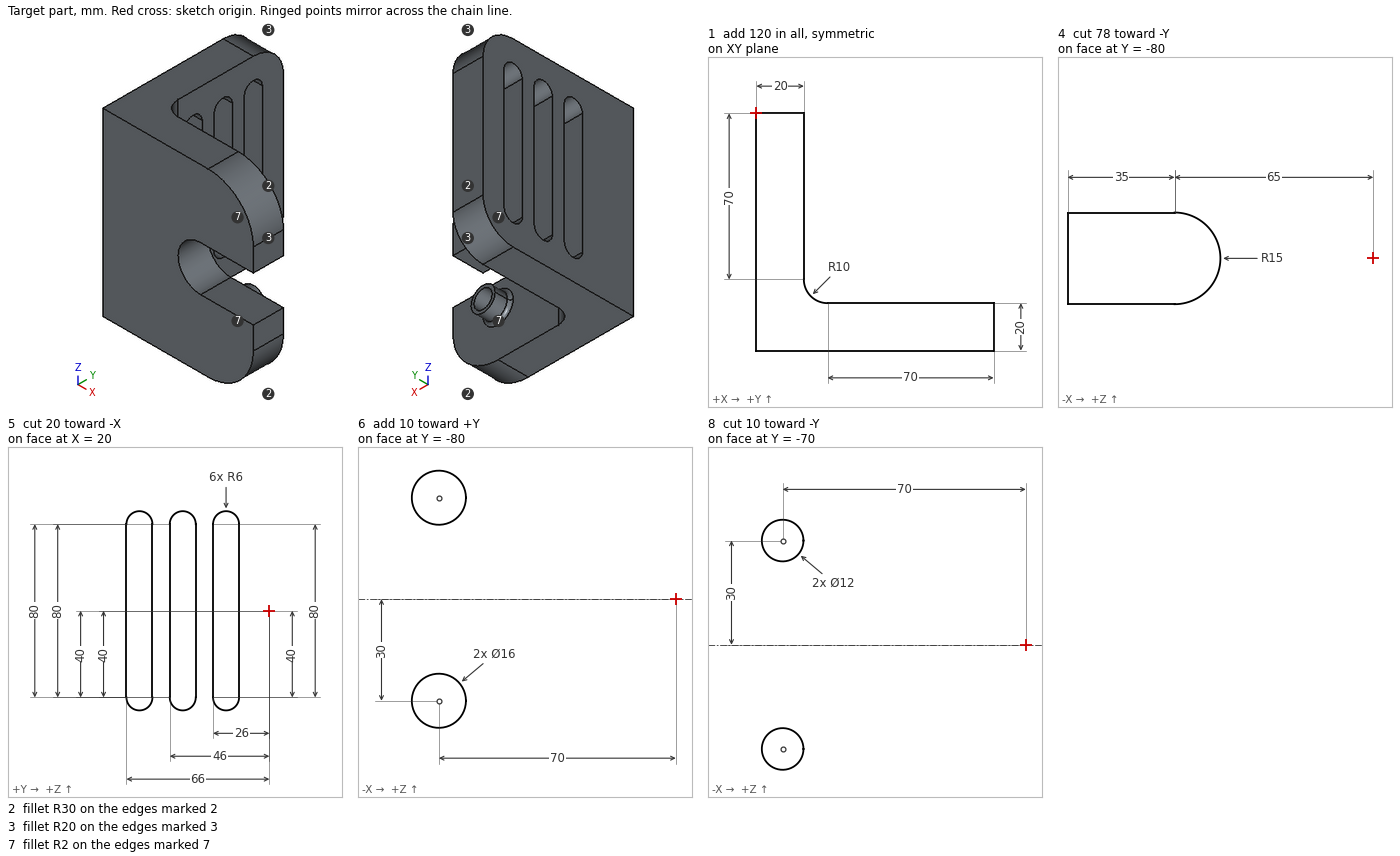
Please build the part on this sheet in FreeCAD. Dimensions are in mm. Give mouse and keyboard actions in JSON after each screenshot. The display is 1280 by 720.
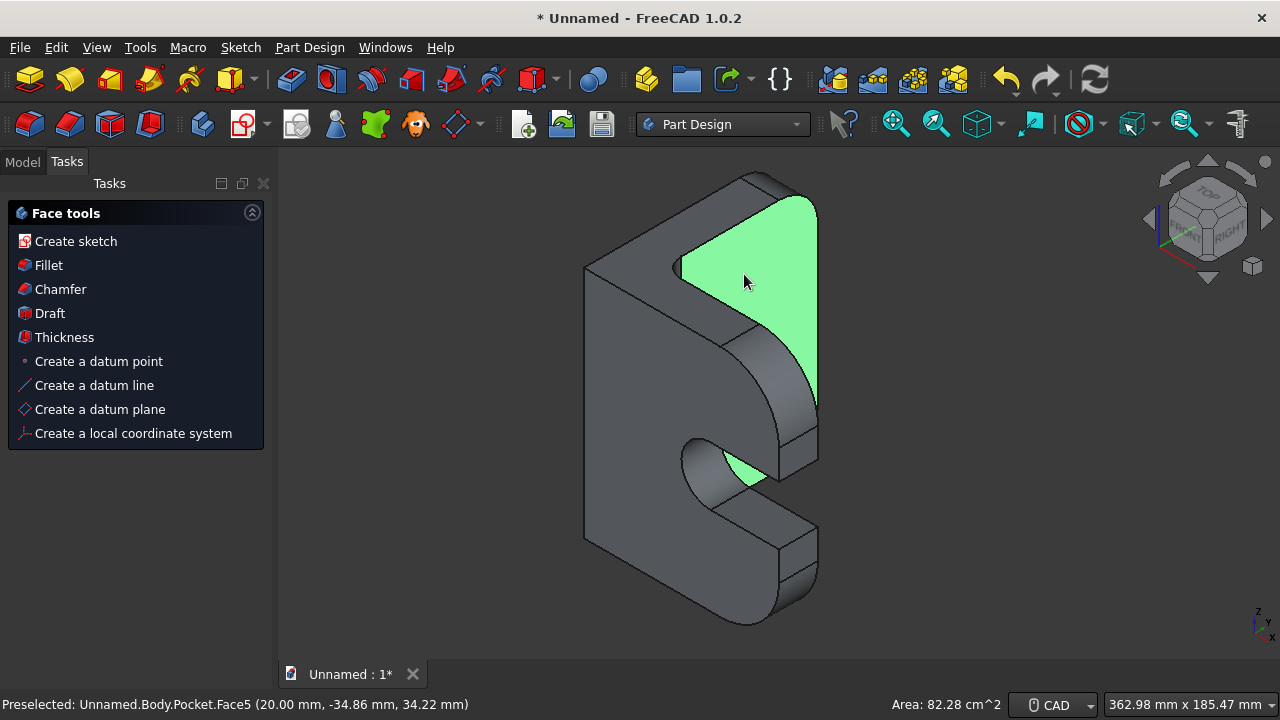
{"action": "left_click", "coordinate": [244, 124]}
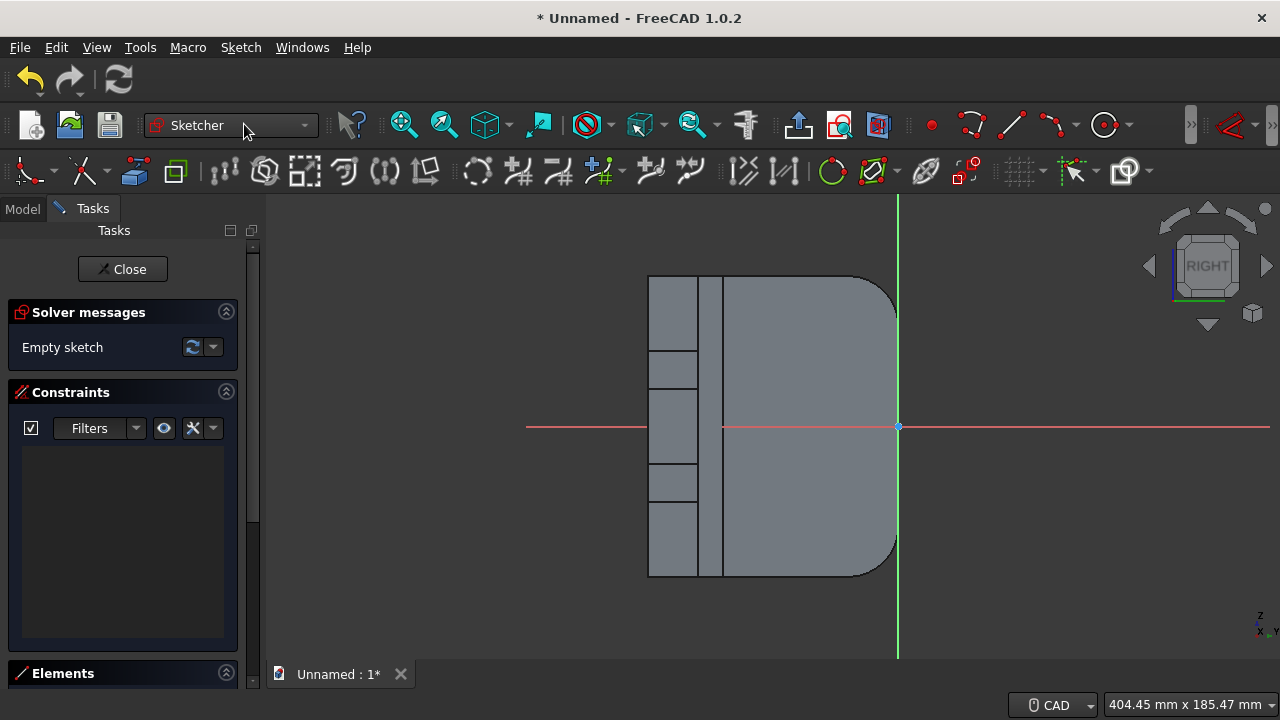
{"action": "left_click", "coordinate": [880, 126]}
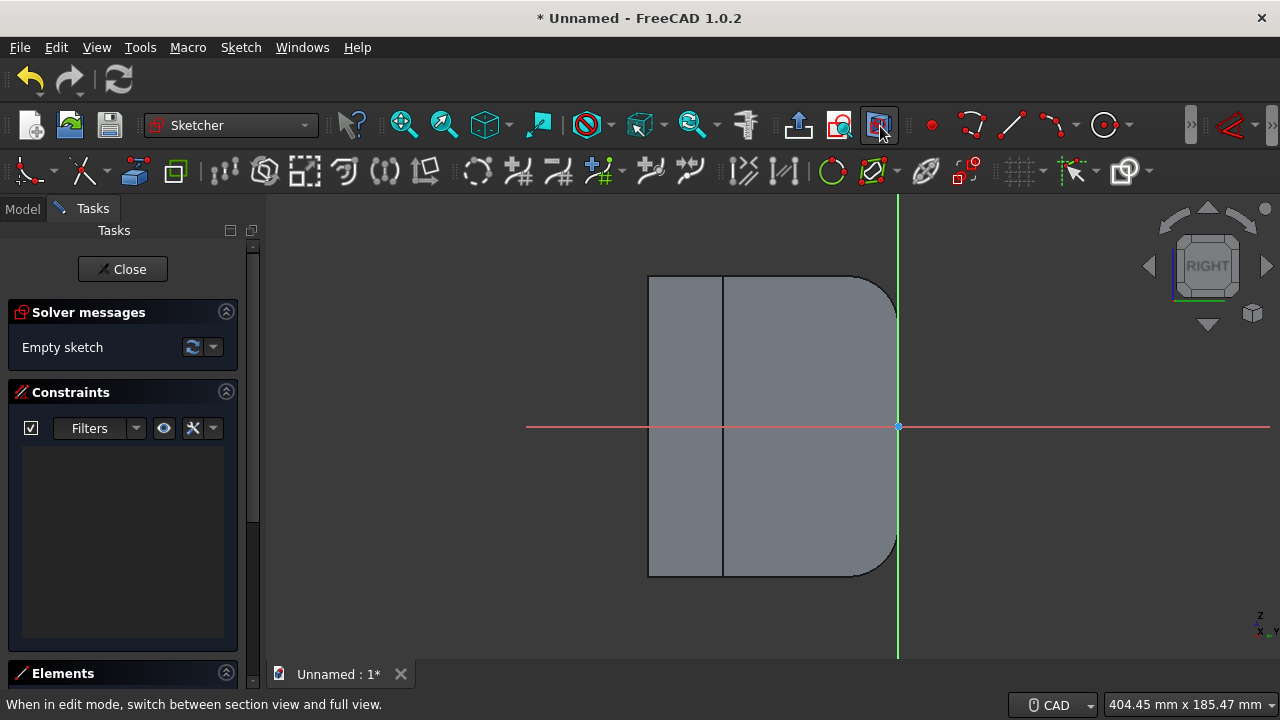
{"action": "key", "text": "g s"}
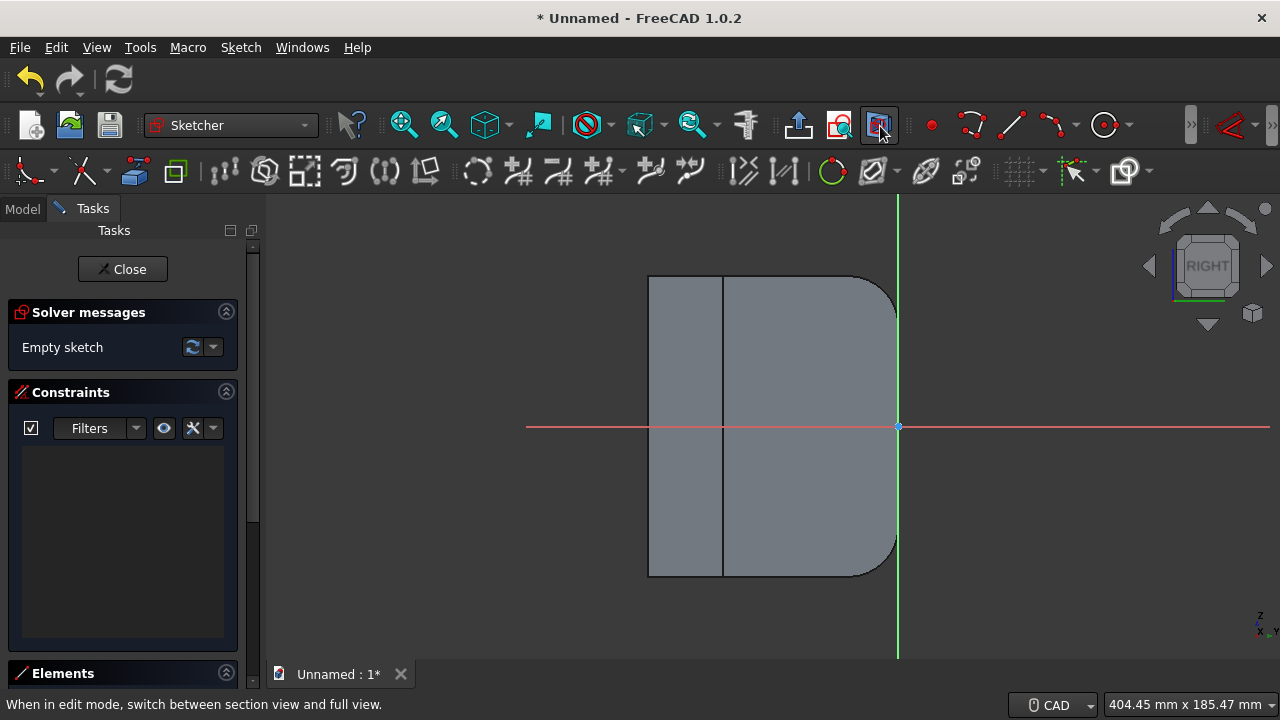
{"action": "scroll", "coordinate": [848, 527], "scroll_direction": "up", "scroll_amount": 3}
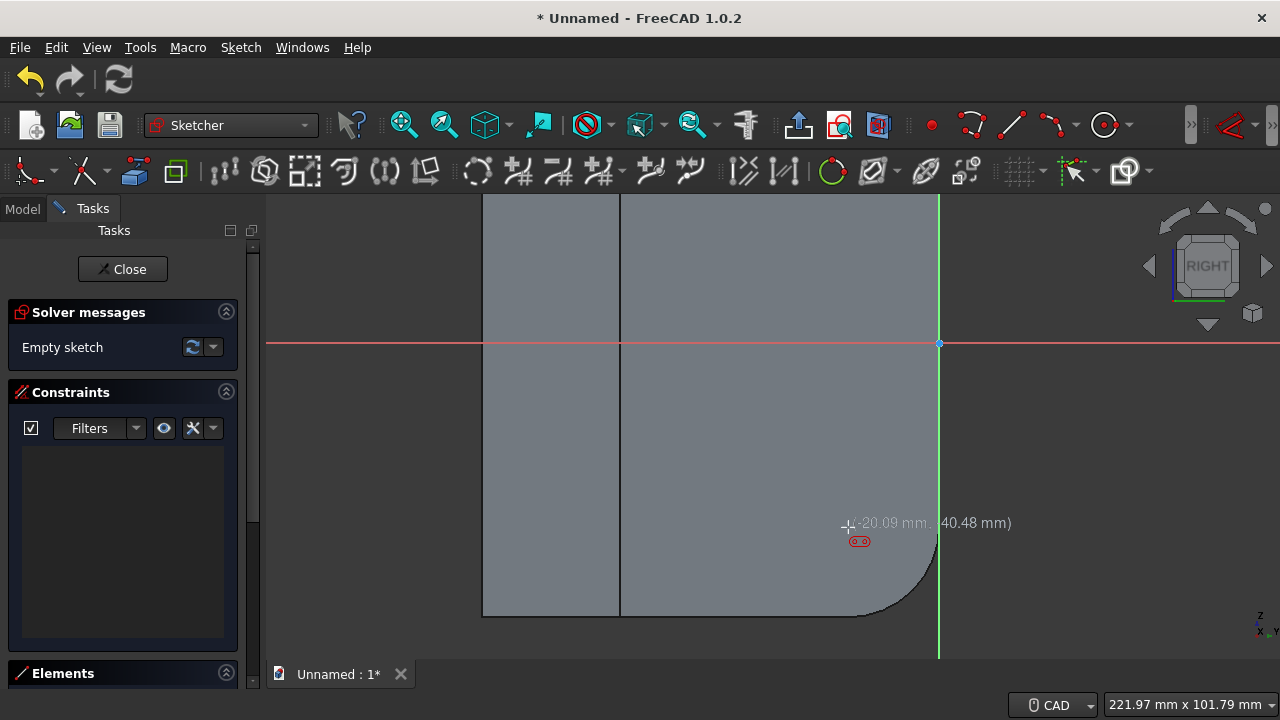
{"action": "left_click", "coordinate": [848, 526]}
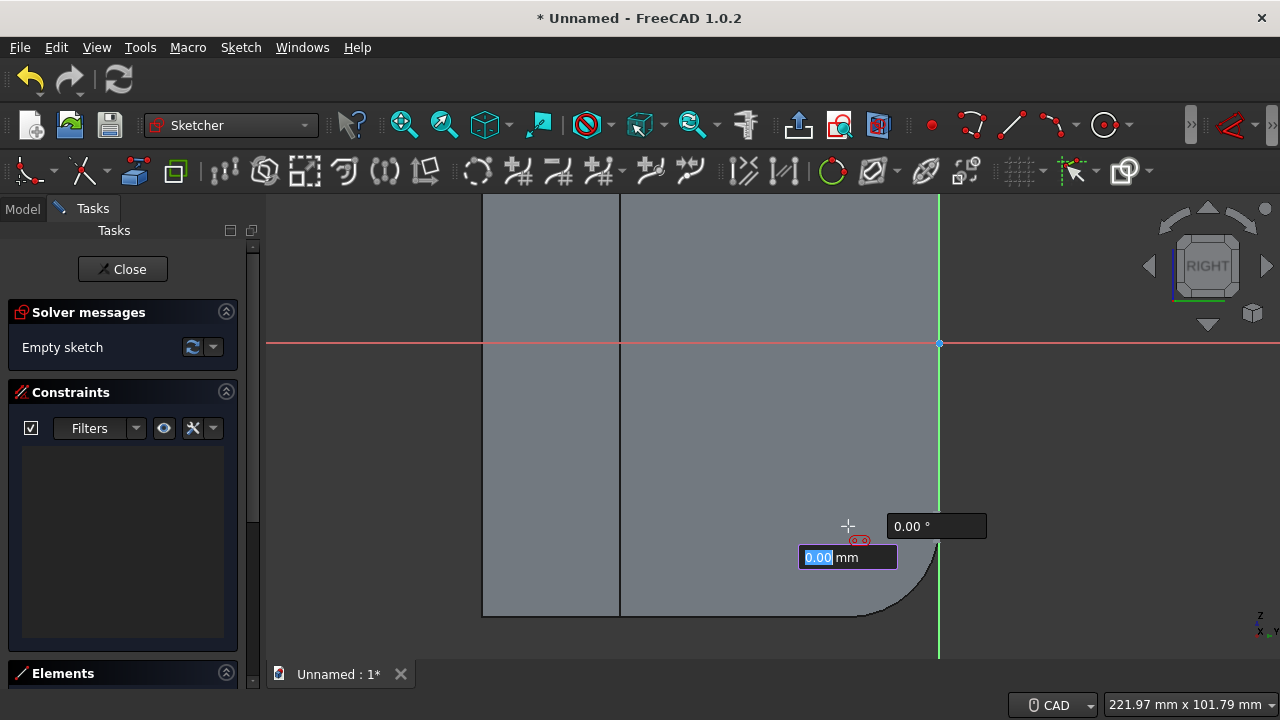
{"action": "scroll", "coordinate": [534, 596], "scroll_direction": "down", "scroll_amount": 2}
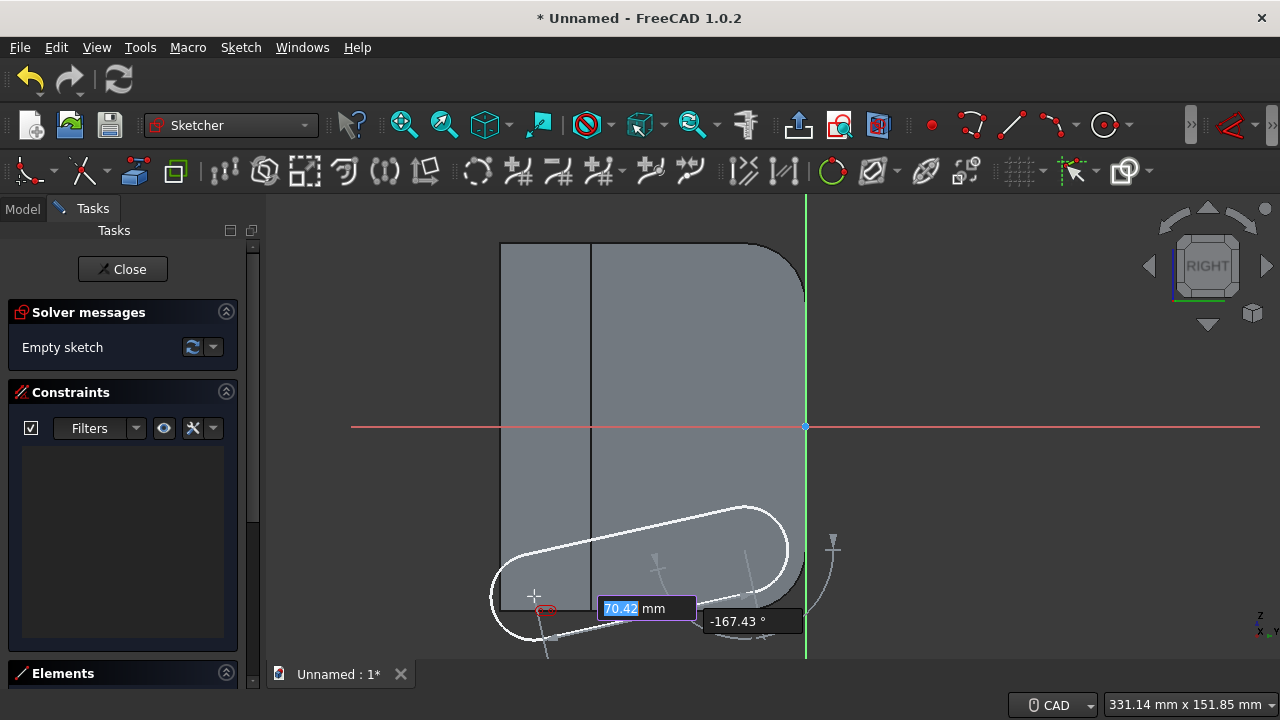
{"action": "left_click", "coordinate": [745, 304]}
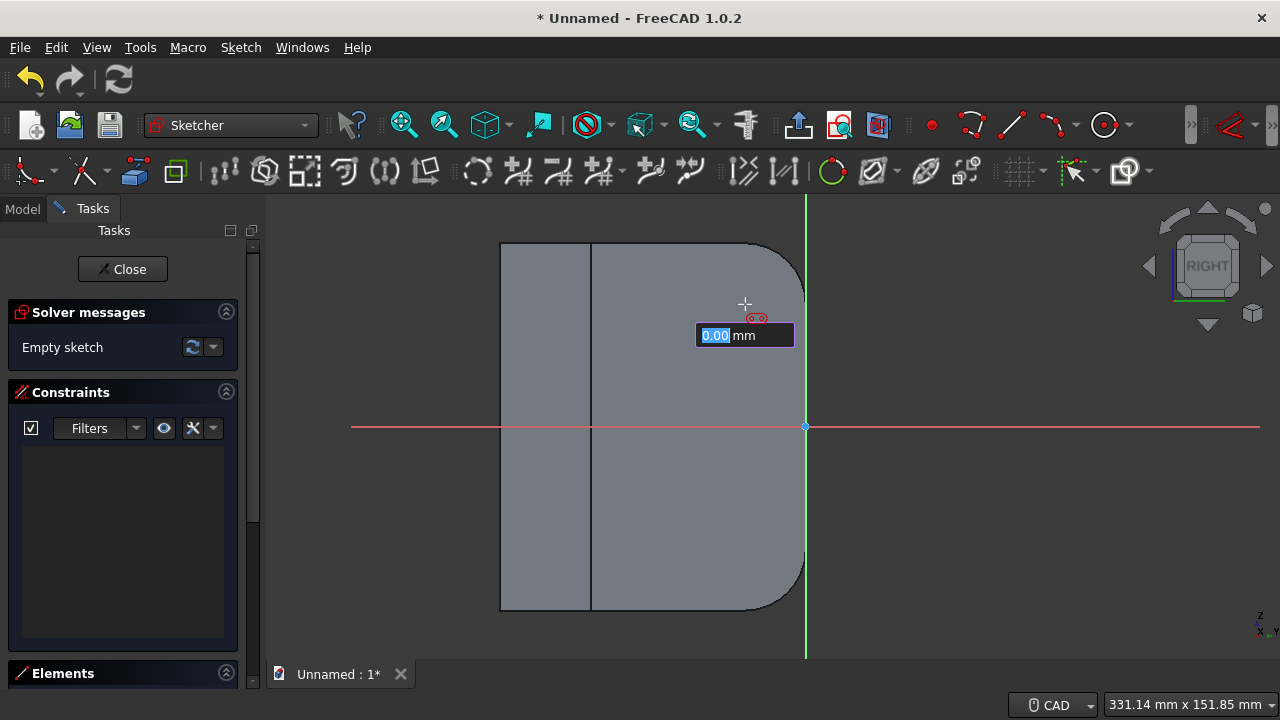
{"action": "left_click", "coordinate": [763, 464]}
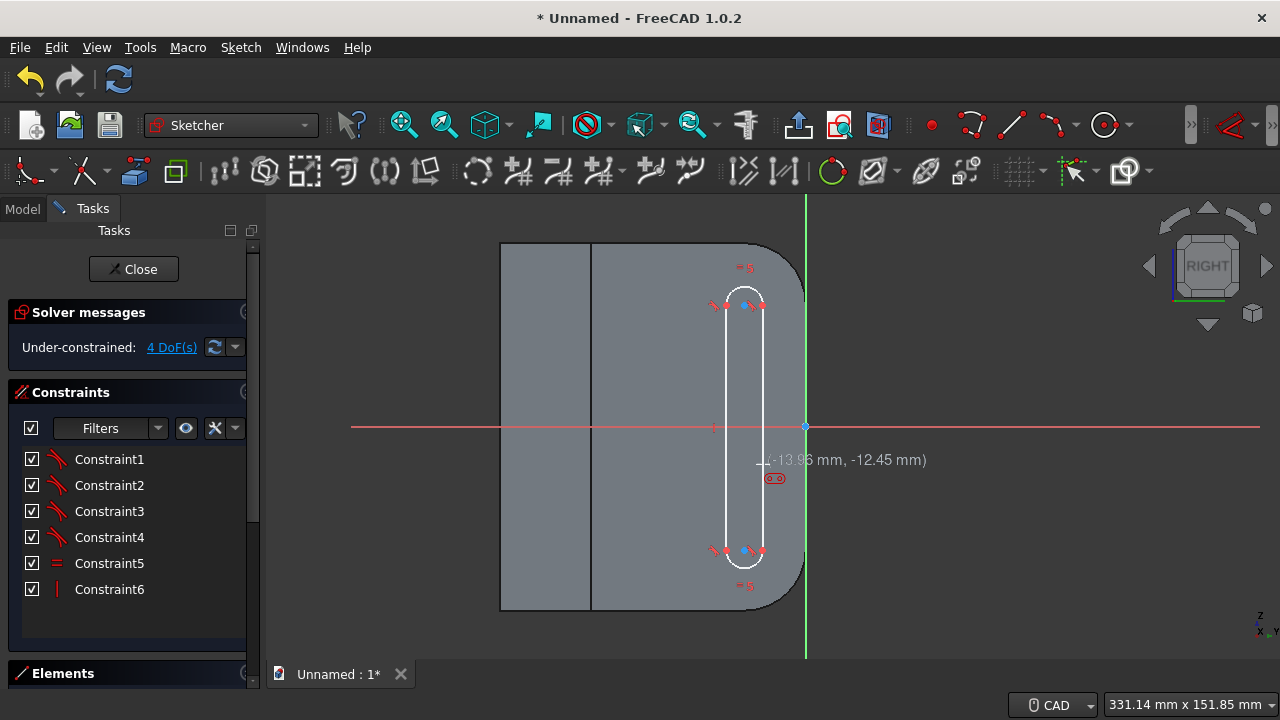
{"action": "scroll", "coordinate": [683, 549], "scroll_direction": "up", "scroll_amount": 2}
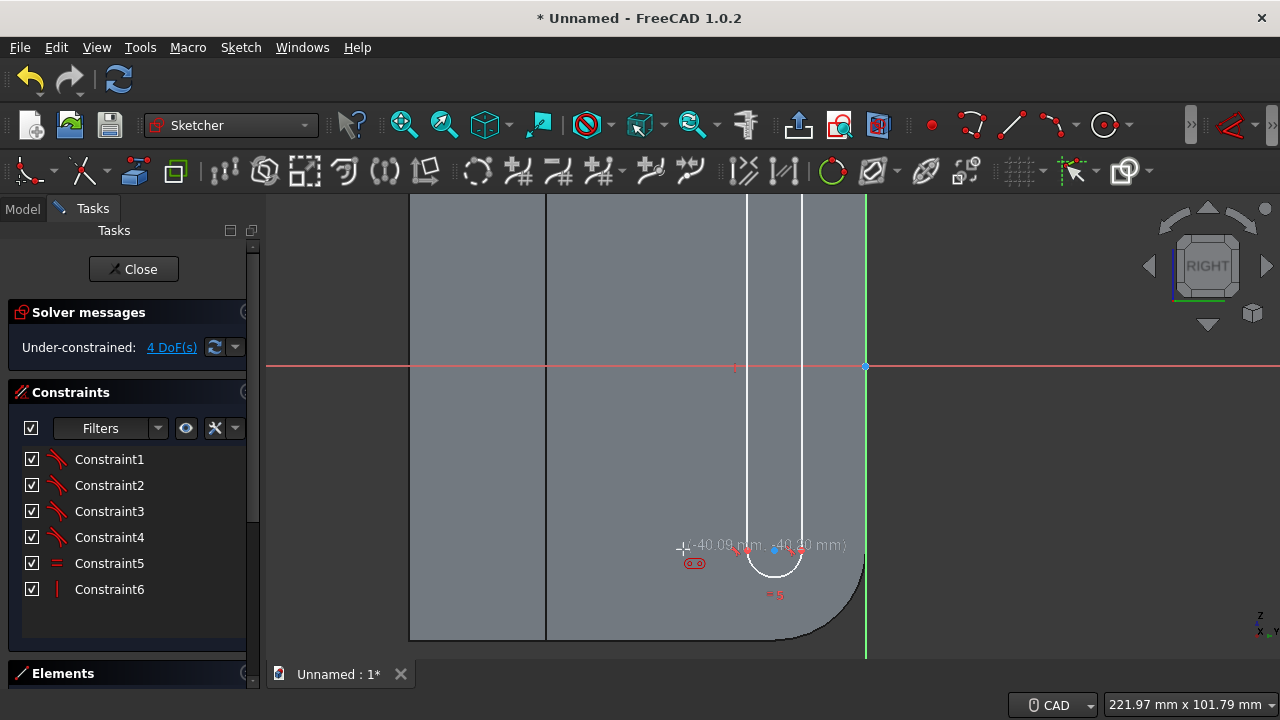
{"action": "left_click", "coordinate": [683, 549]}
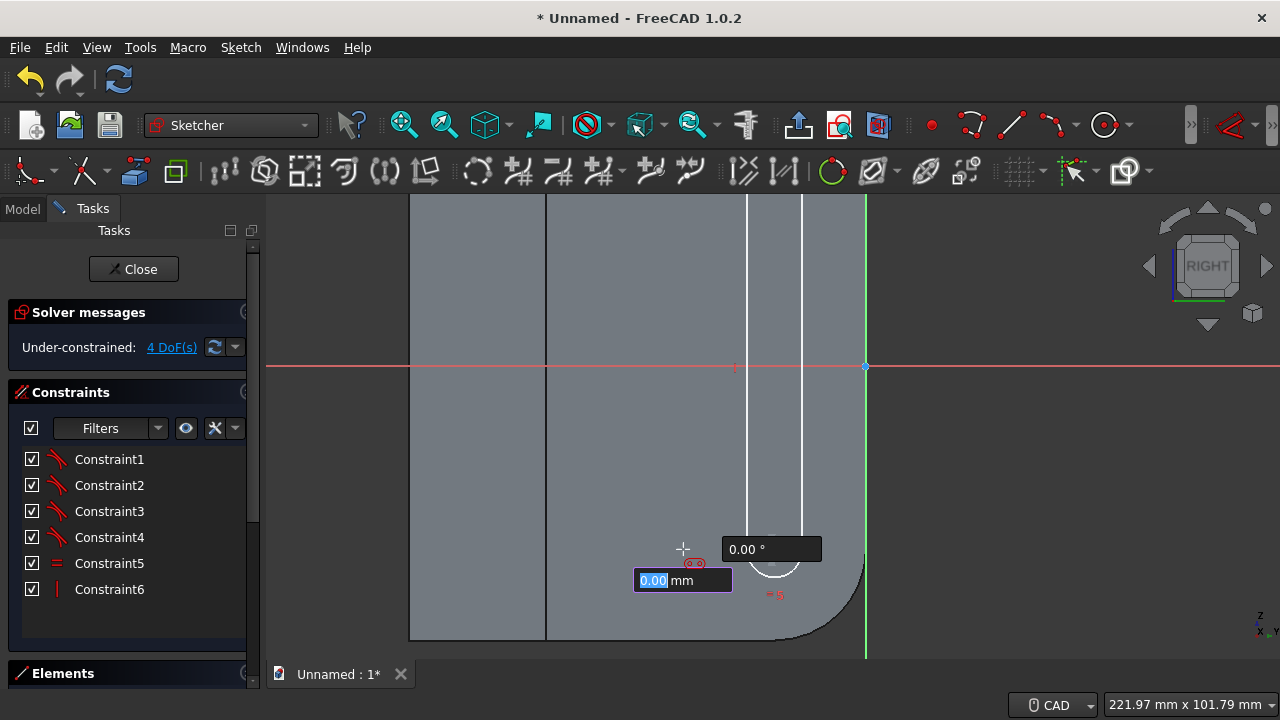
{"action": "scroll", "coordinate": [683, 549], "scroll_direction": "down", "scroll_amount": 2}